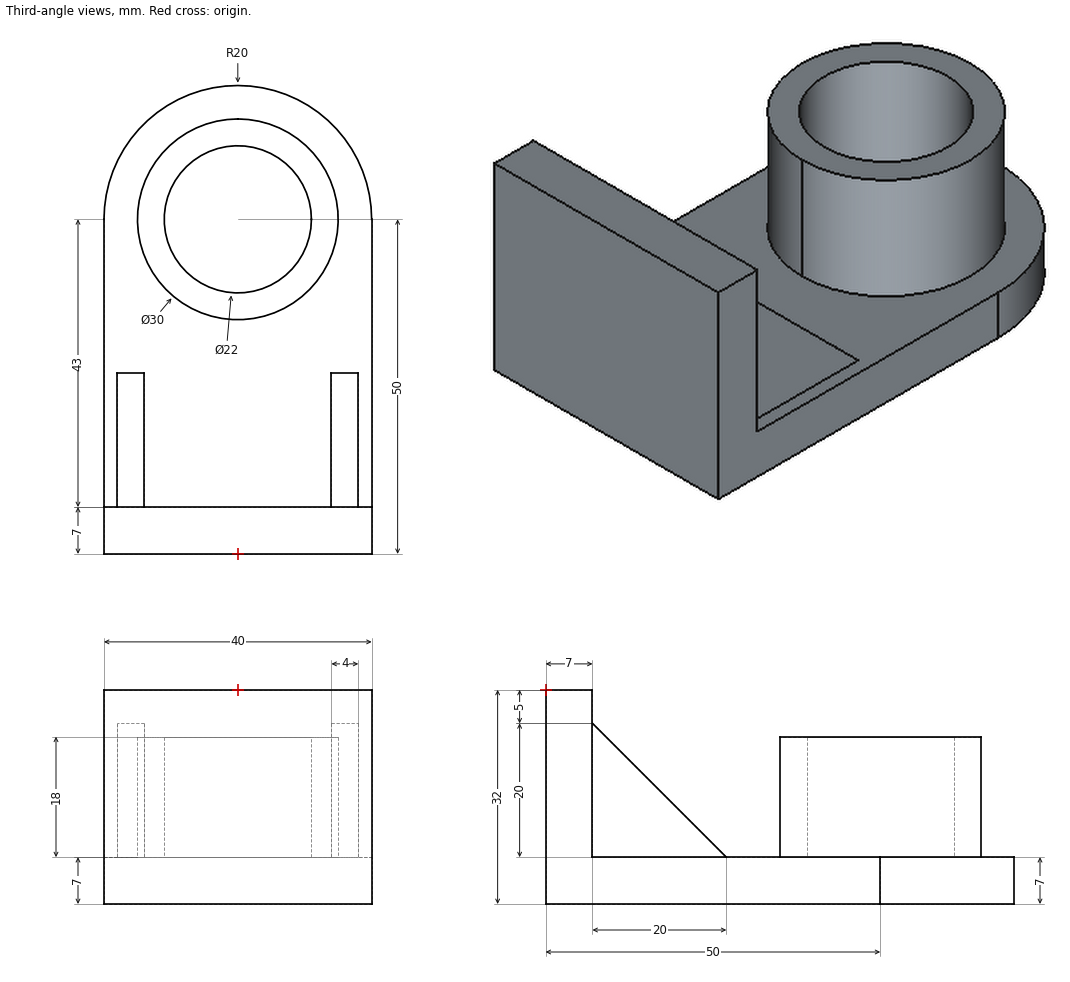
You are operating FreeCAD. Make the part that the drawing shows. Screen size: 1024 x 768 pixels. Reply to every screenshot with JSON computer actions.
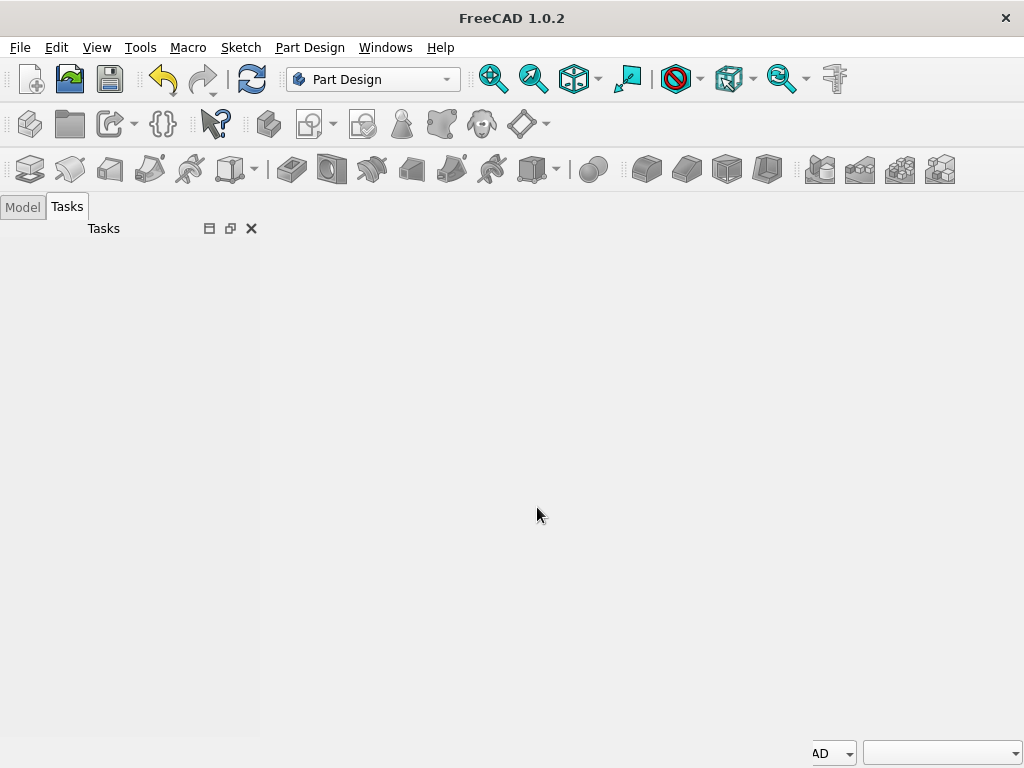
{"action": "left_click", "coordinate": [30, 80]}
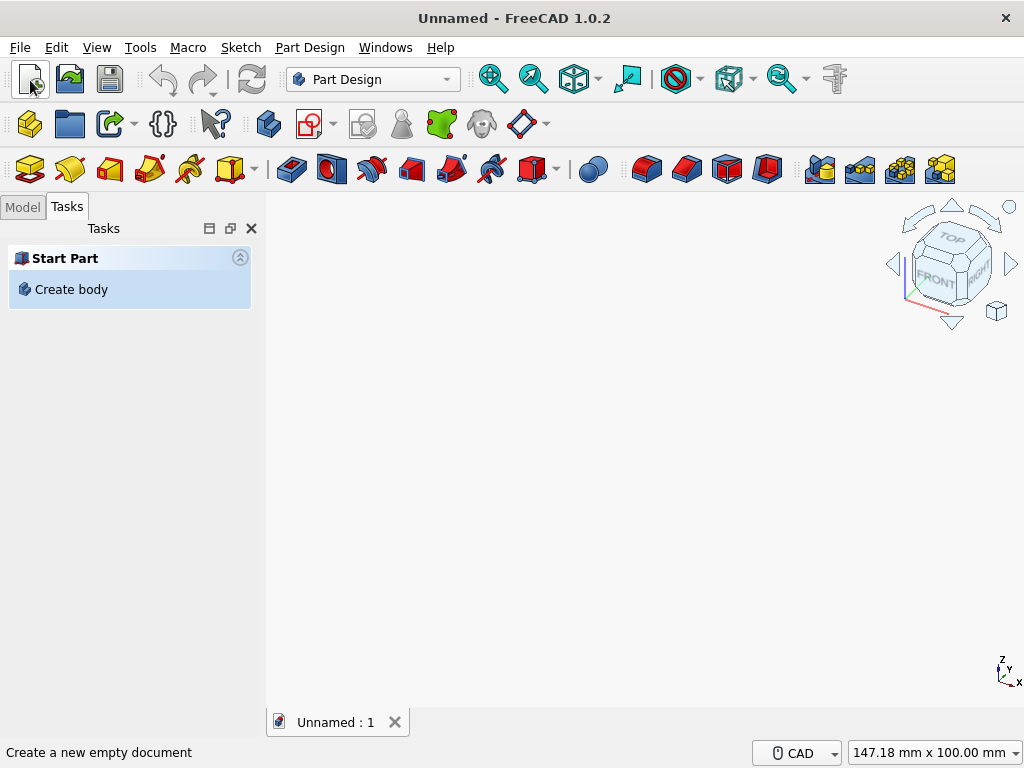
{"action": "left_click", "coordinate": [310, 124]}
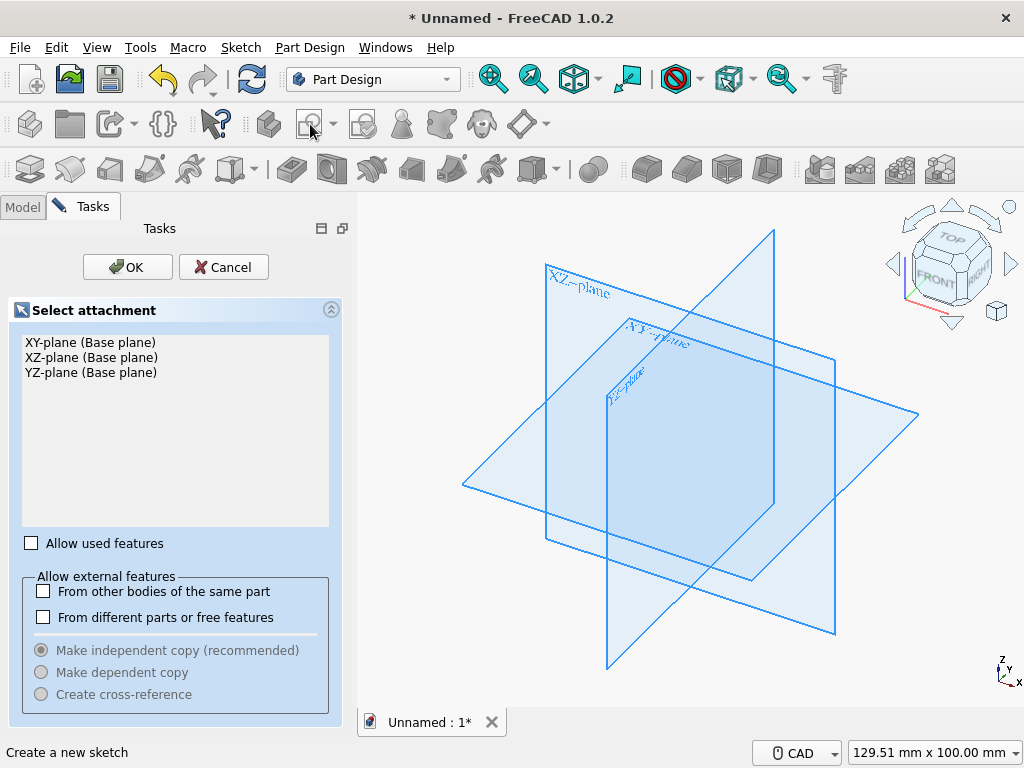
{"action": "left_click", "coordinate": [82, 372]}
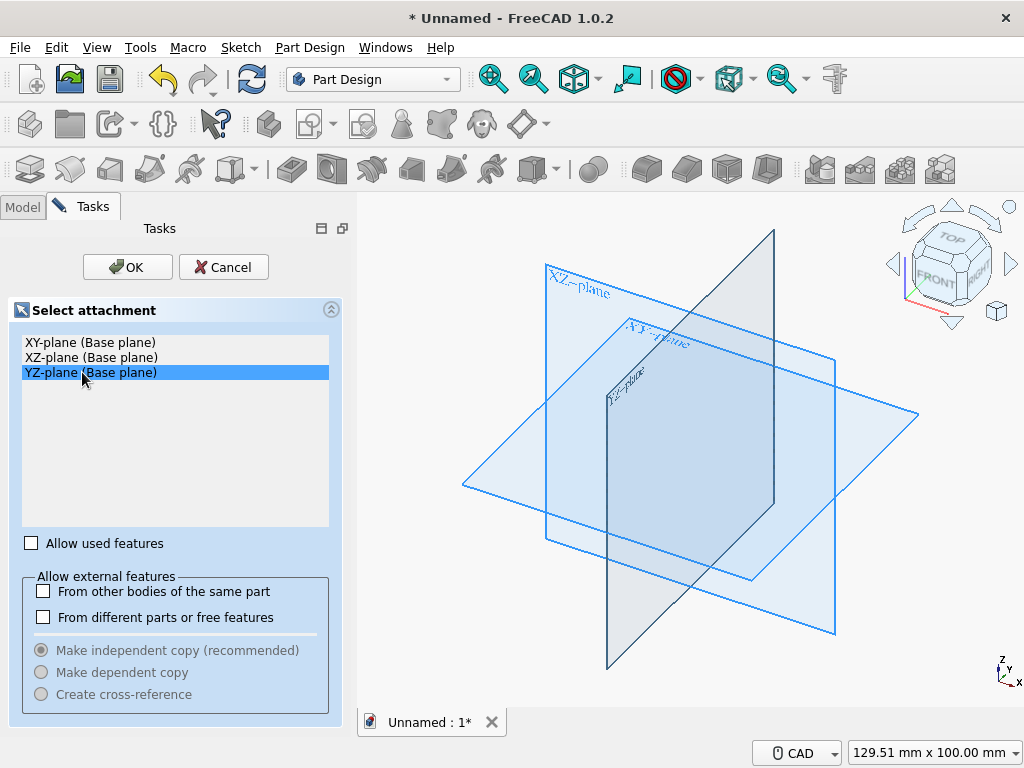
{"action": "left_click", "coordinate": [128, 267]}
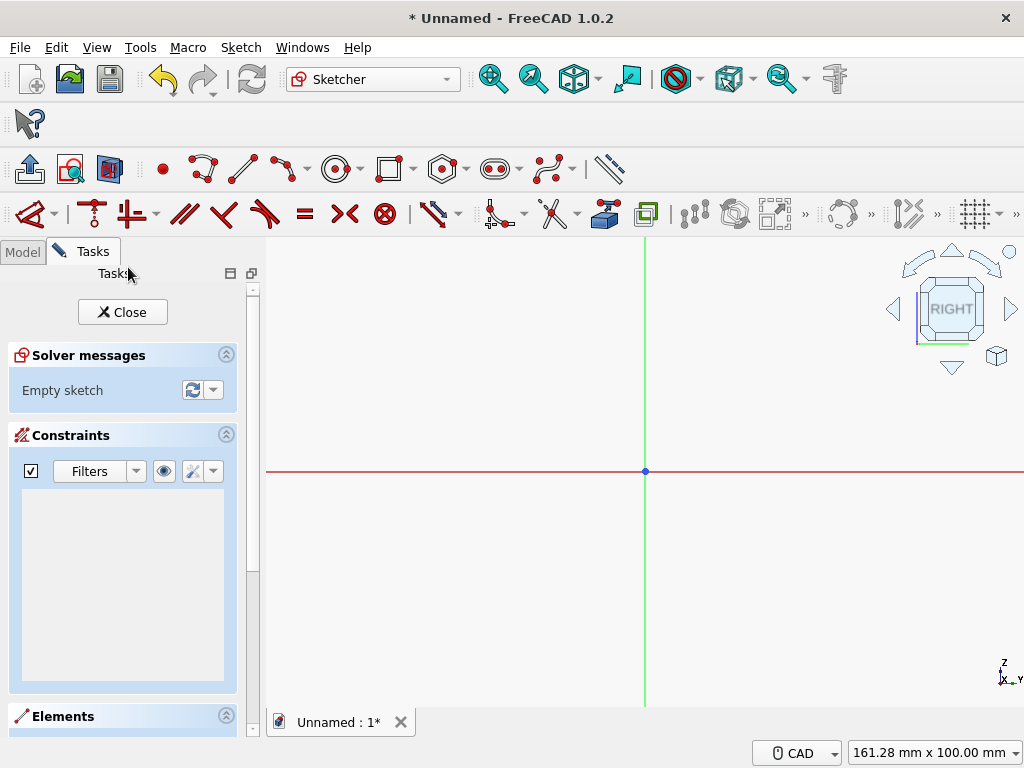
{"action": "scroll", "coordinate": [576, 472], "scroll_direction": "down", "scroll_amount": 5}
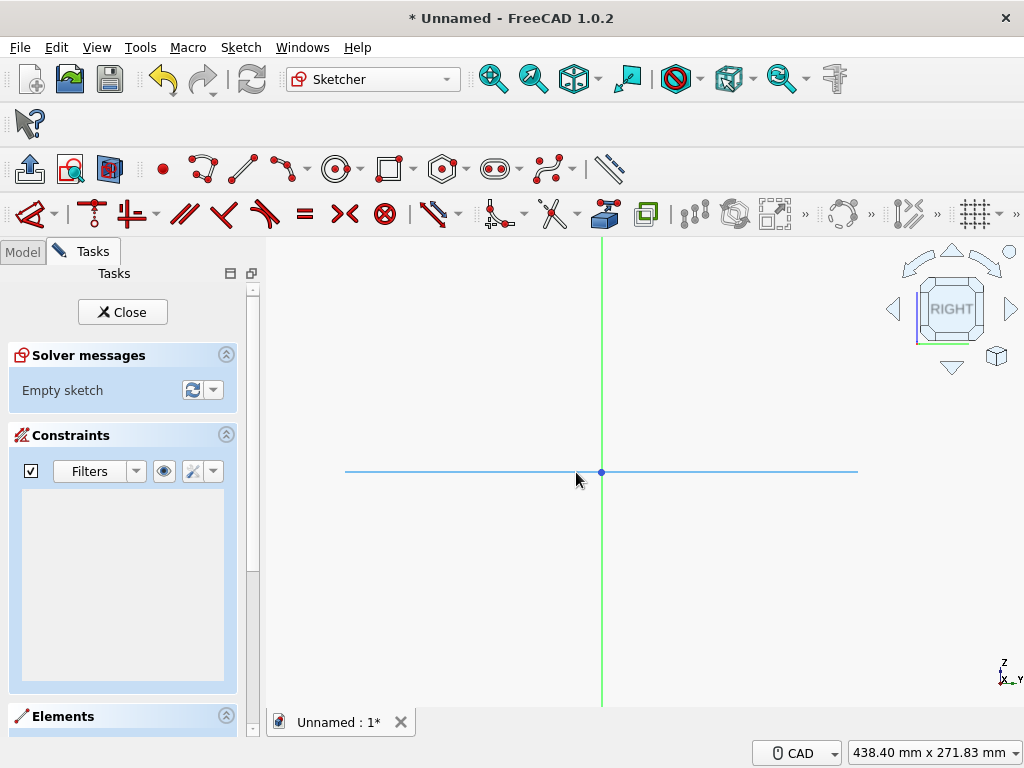
{"action": "scroll", "coordinate": [662, 507], "scroll_direction": "up", "scroll_amount": 8}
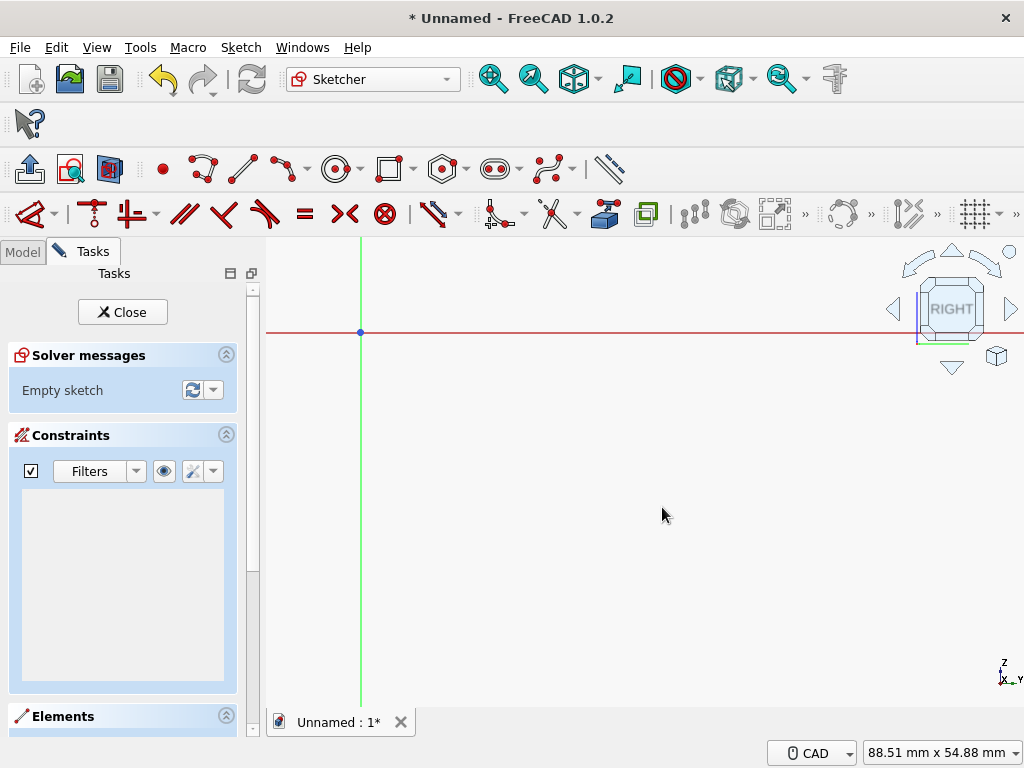
{"action": "left_click", "coordinate": [204, 170]}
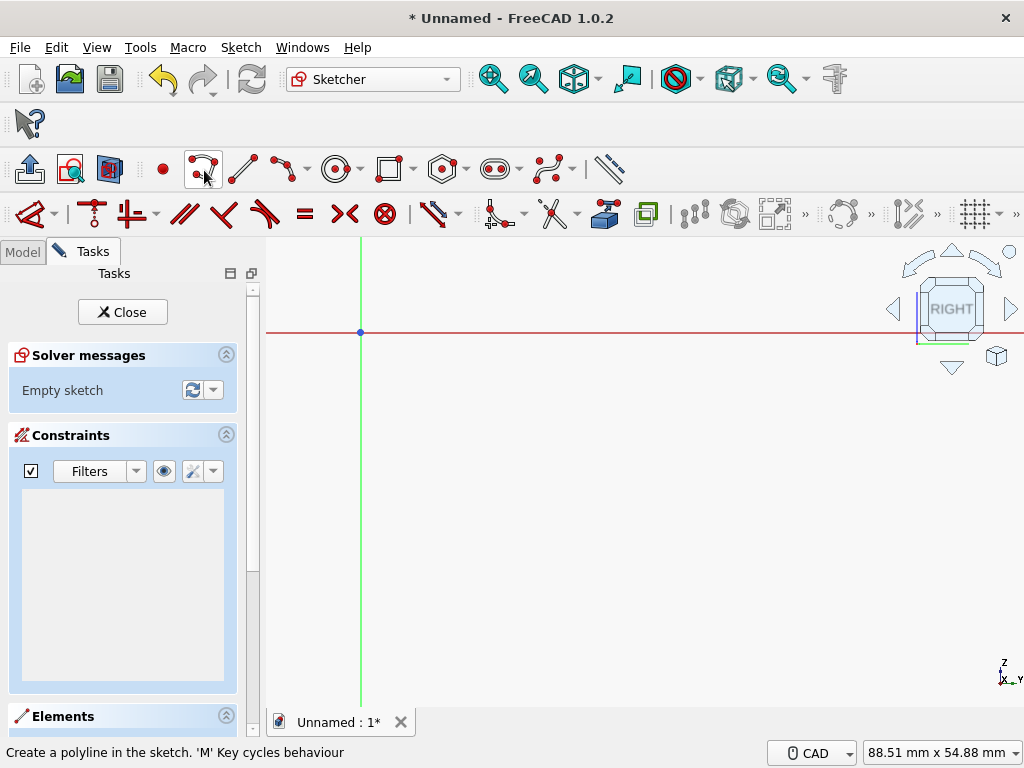
{"action": "left_click", "coordinate": [361, 333]}
{"action": "left_click", "coordinate": [370, 607]}
{"action": "left_click", "coordinate": [789, 607]}
{"action": "left_click", "coordinate": [789, 547]}
{"action": "left_click", "coordinate": [421, 547]}
{"action": "left_click", "coordinate": [421, 342]}
{"action": "left_click", "coordinate": [361, 333]}
{"action": "key", "text": "Escape"}
{"action": "key", "text": "Escape"}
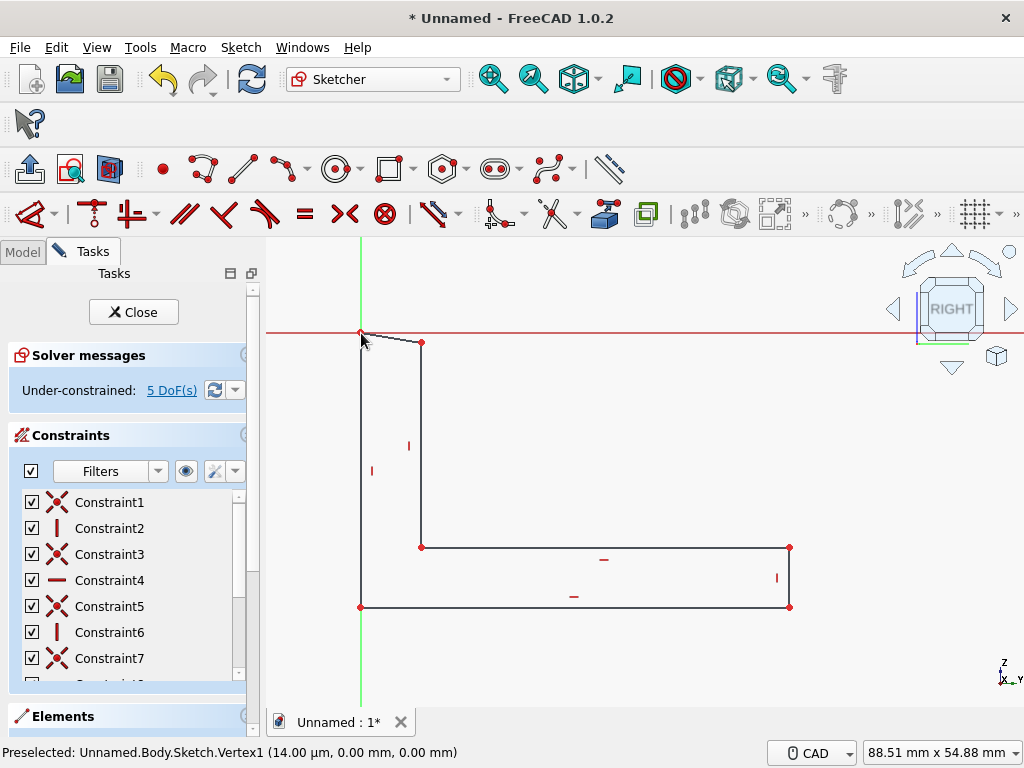
{"action": "left_click", "coordinate": [379, 336]}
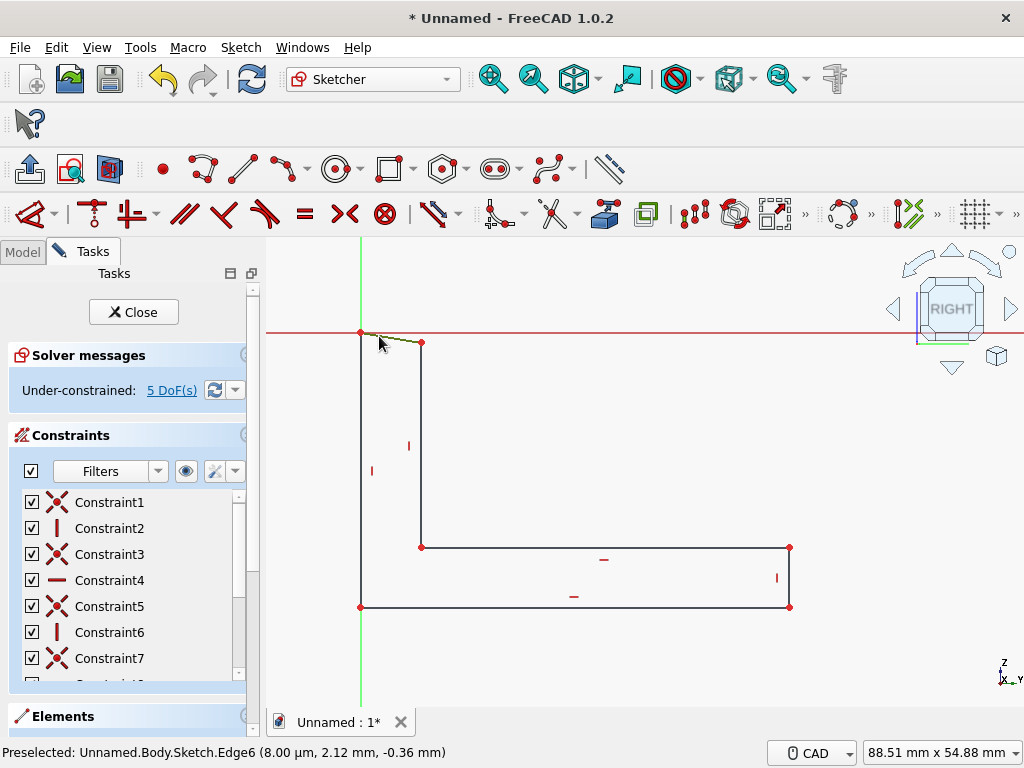
{"action": "key", "text": "h"}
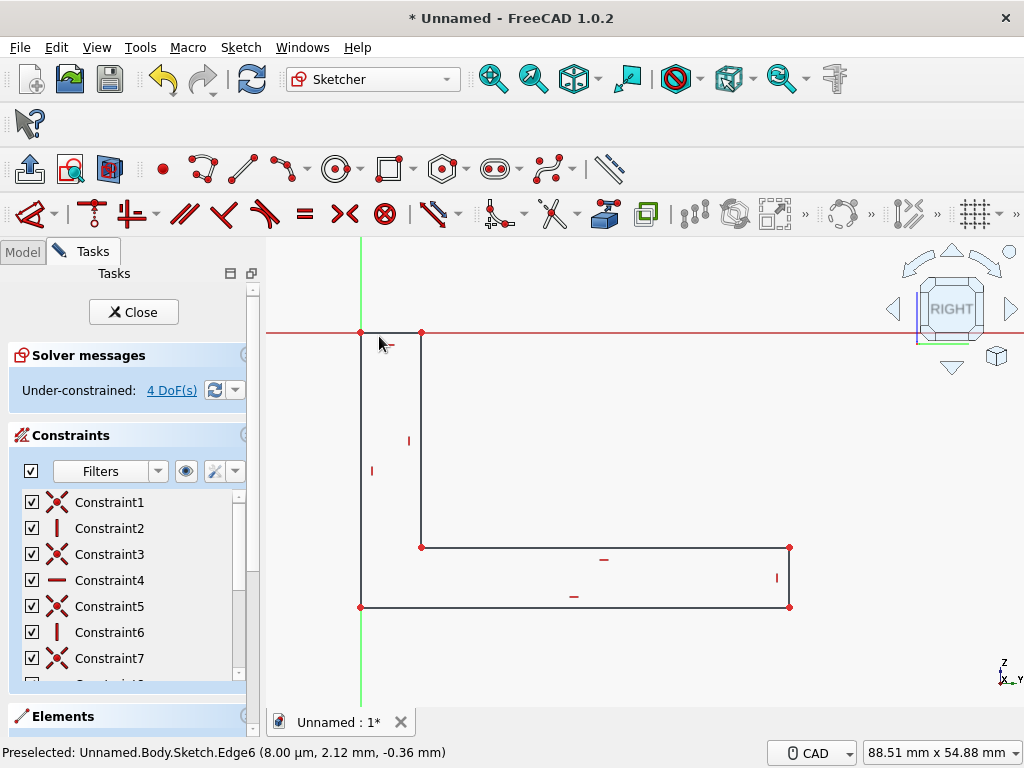
{"action": "left_click", "coordinate": [30, 214]}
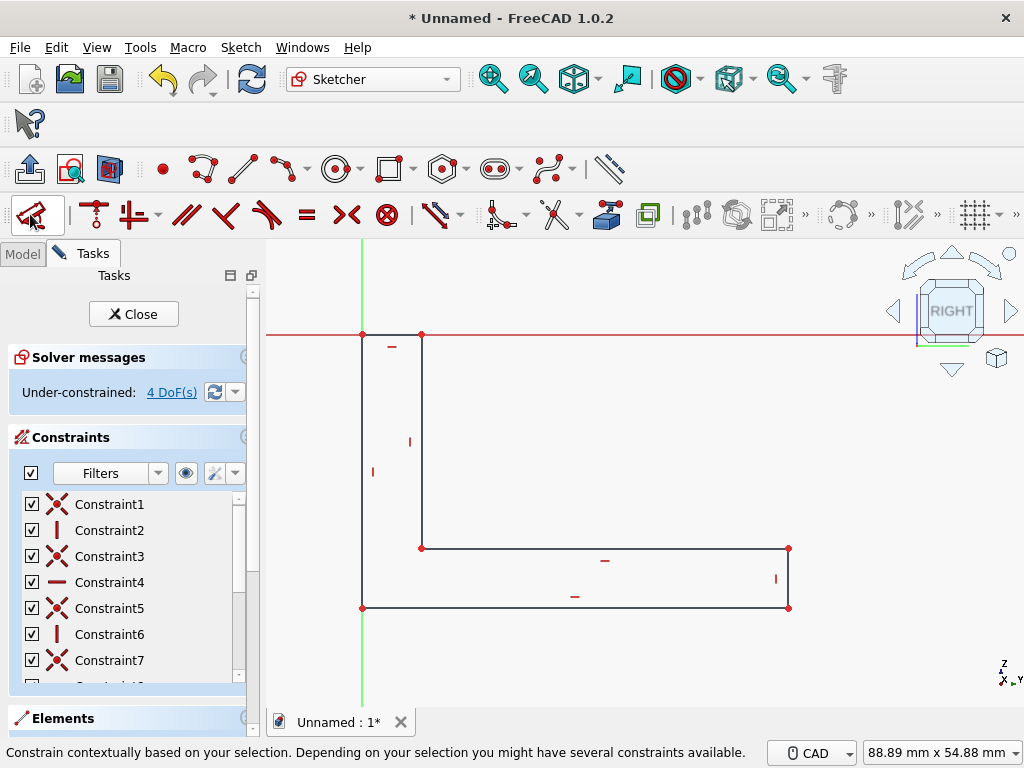
{"action": "left_click", "coordinate": [788, 590]}
{"action": "left_click", "coordinate": [822, 579]}